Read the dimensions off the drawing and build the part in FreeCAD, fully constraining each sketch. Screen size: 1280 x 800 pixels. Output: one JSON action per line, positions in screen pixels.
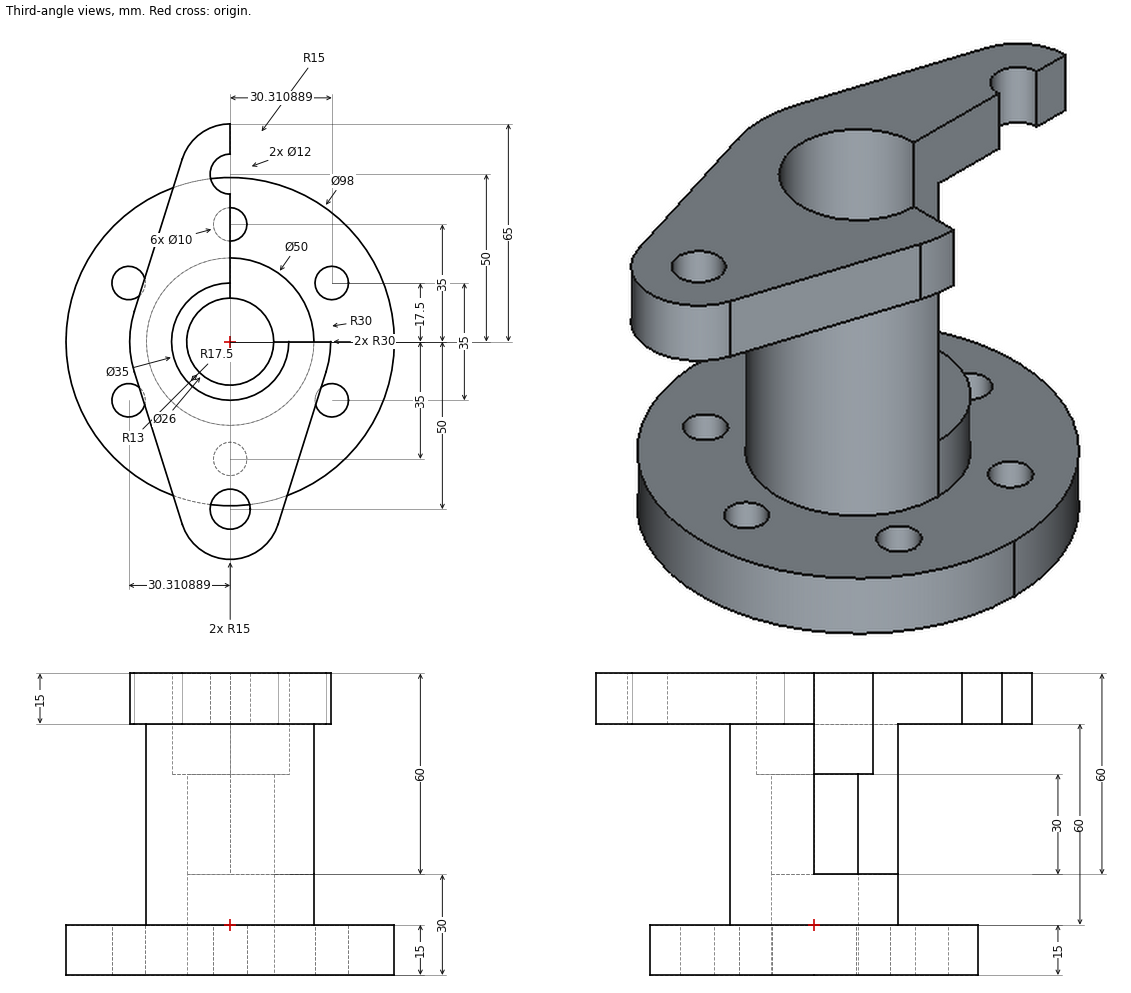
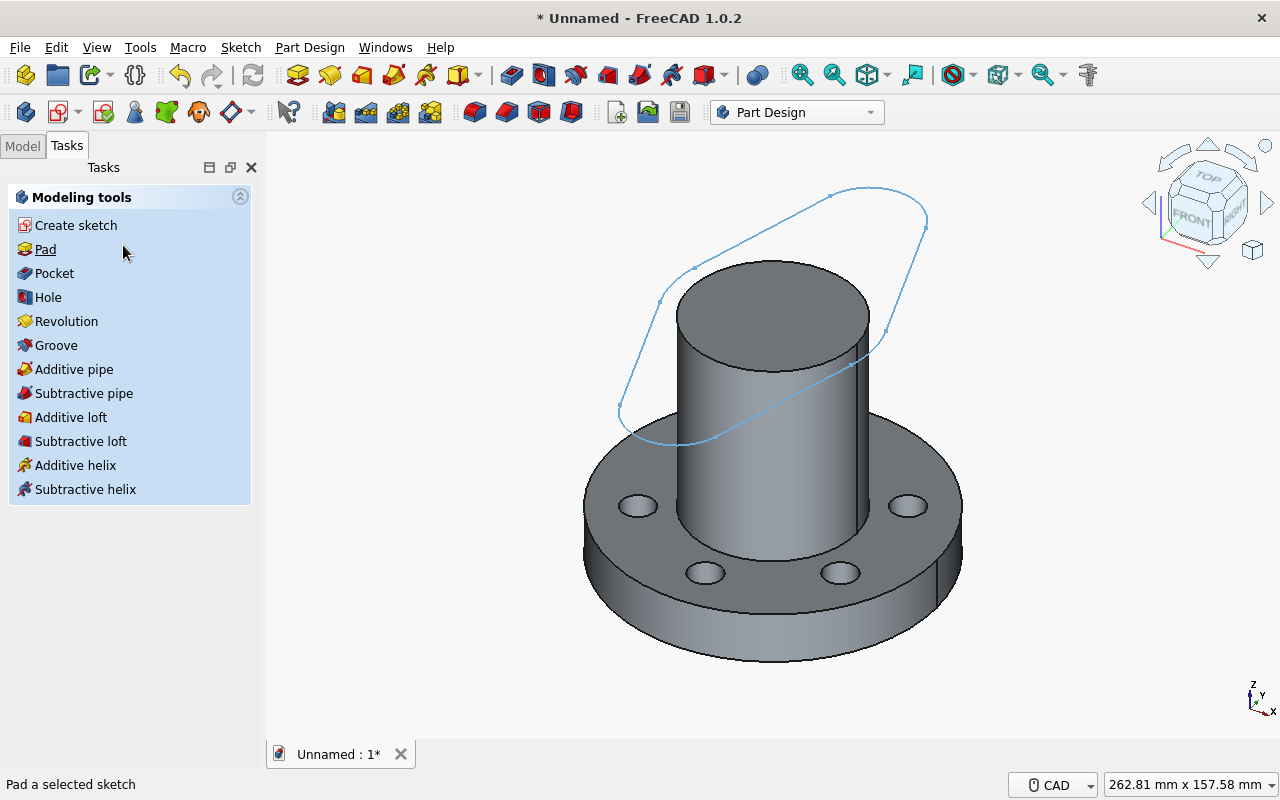
{"action": "left_click", "coordinate": [298, 76]}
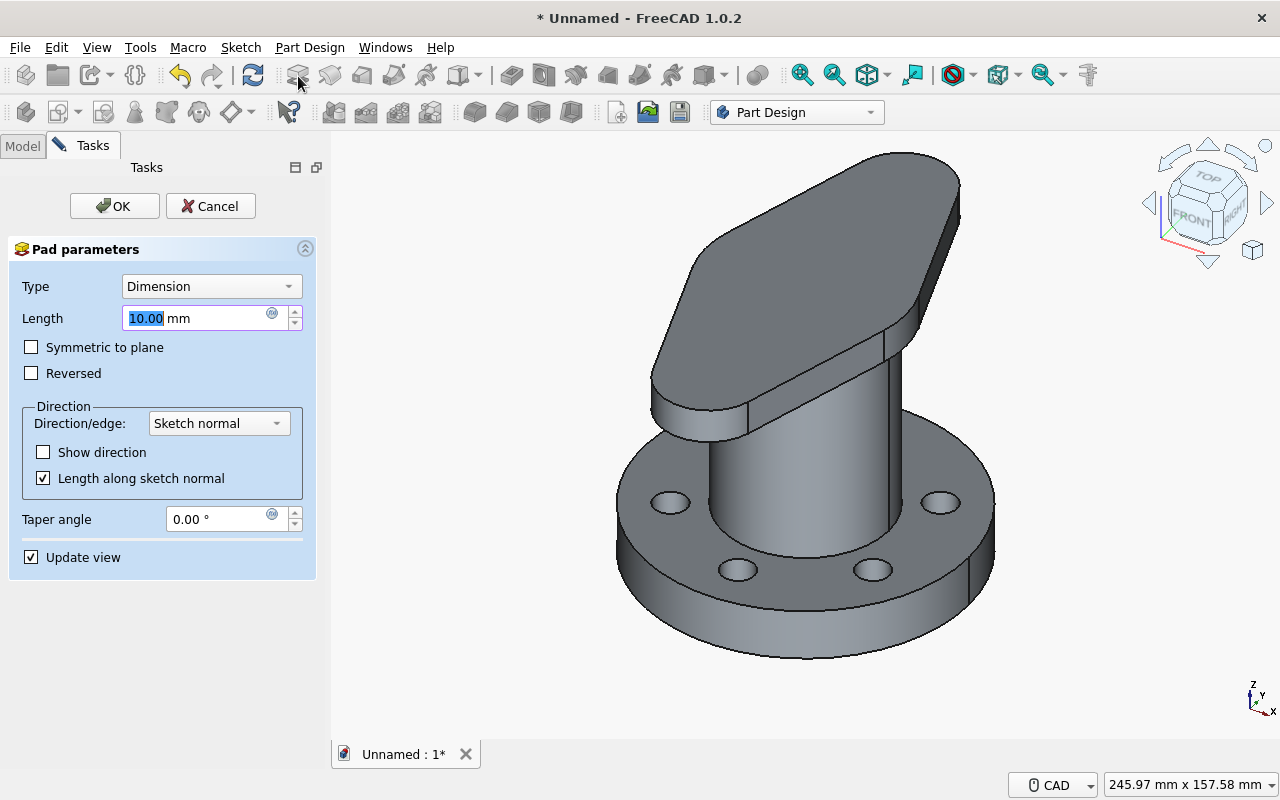
{"action": "type", "text": "15"}
{"action": "key", "text": "Tab"}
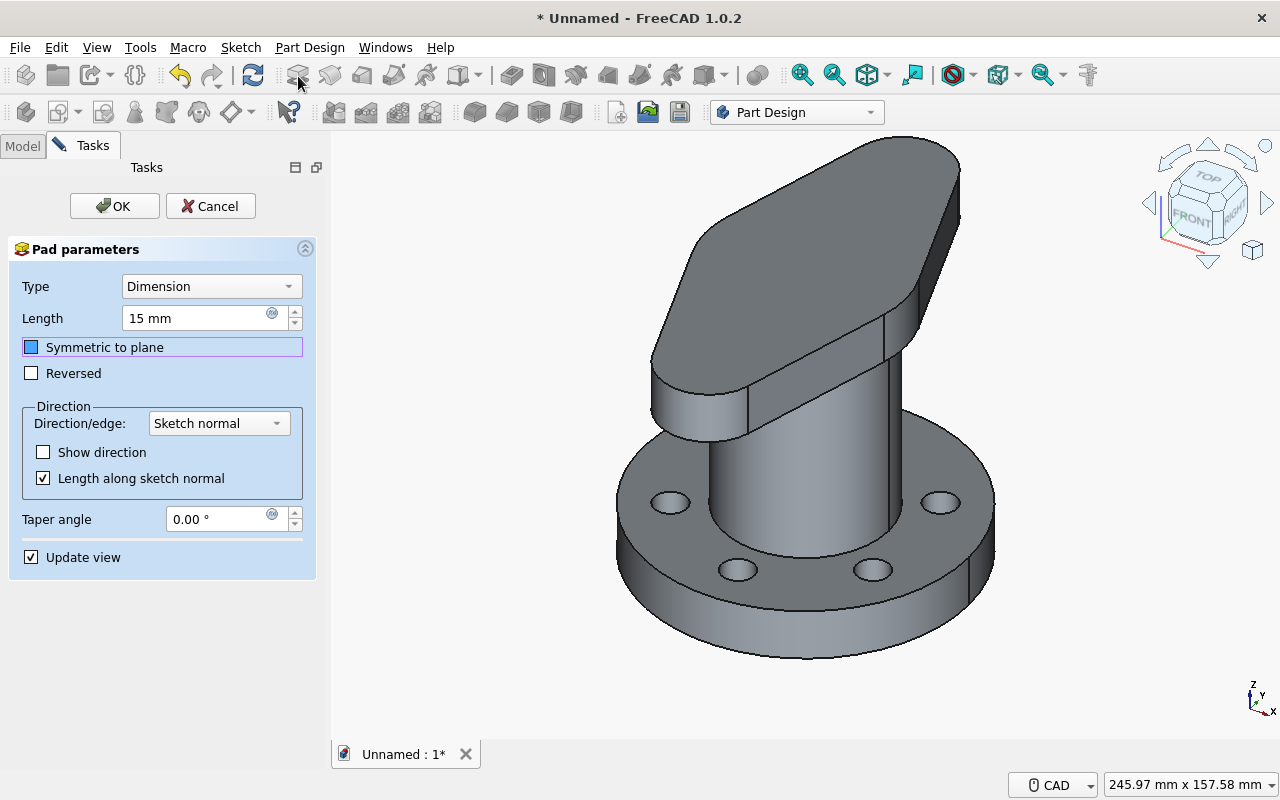
{"action": "left_click", "coordinate": [115, 206]}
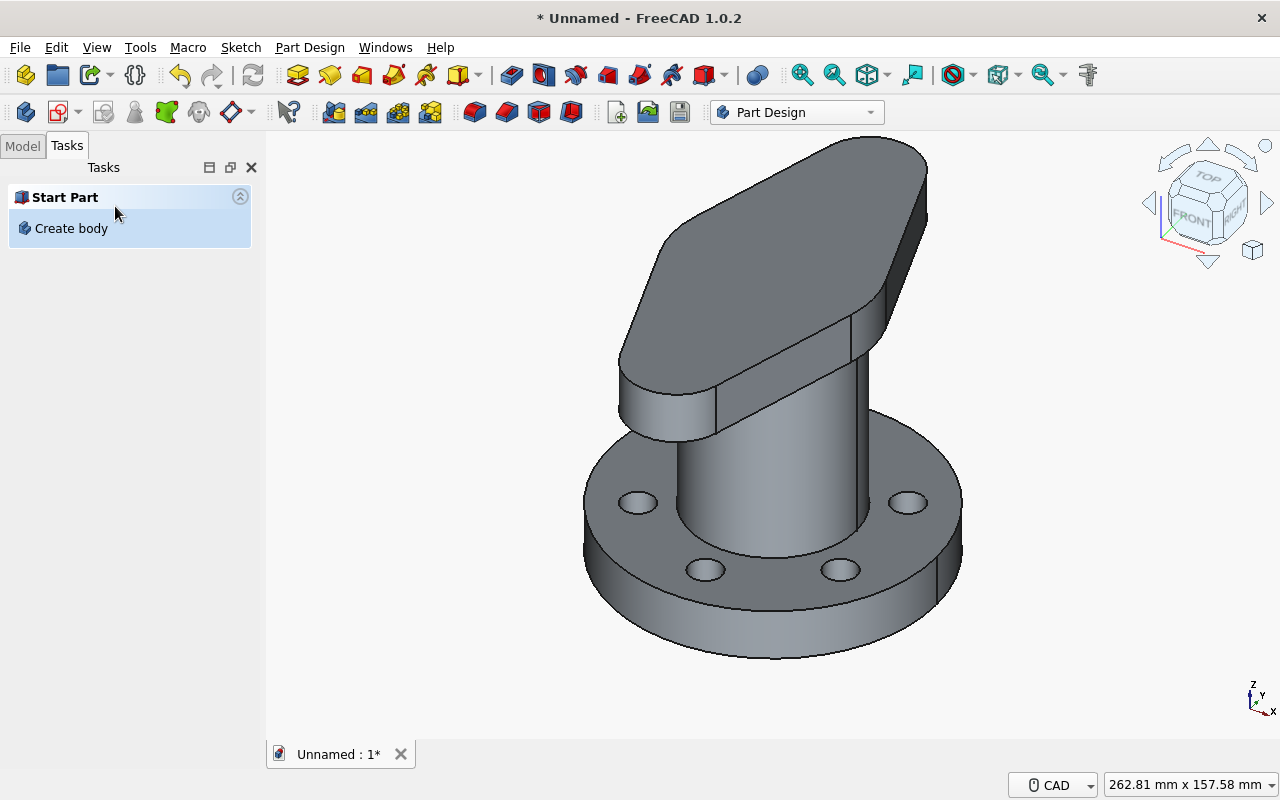
{"action": "left_click", "coordinate": [804, 76]}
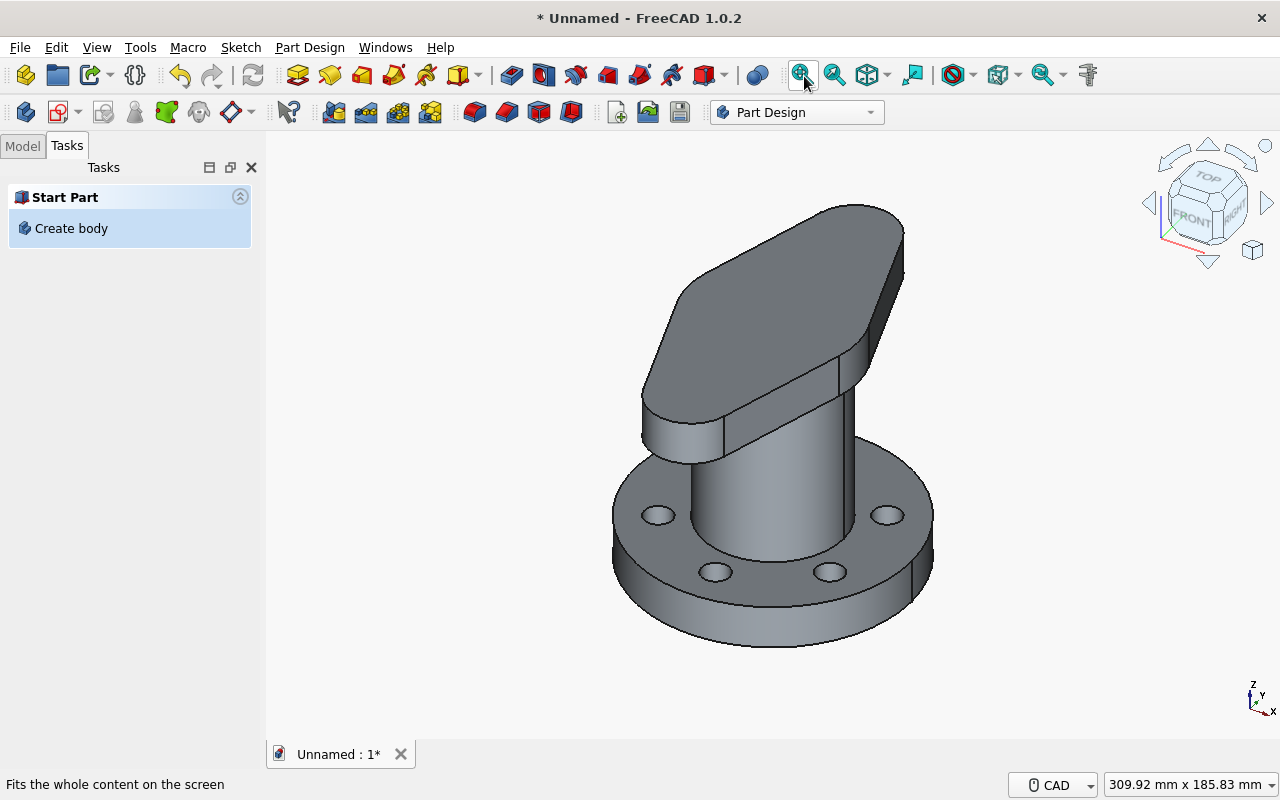
{"action": "left_click", "coordinate": [23, 145]}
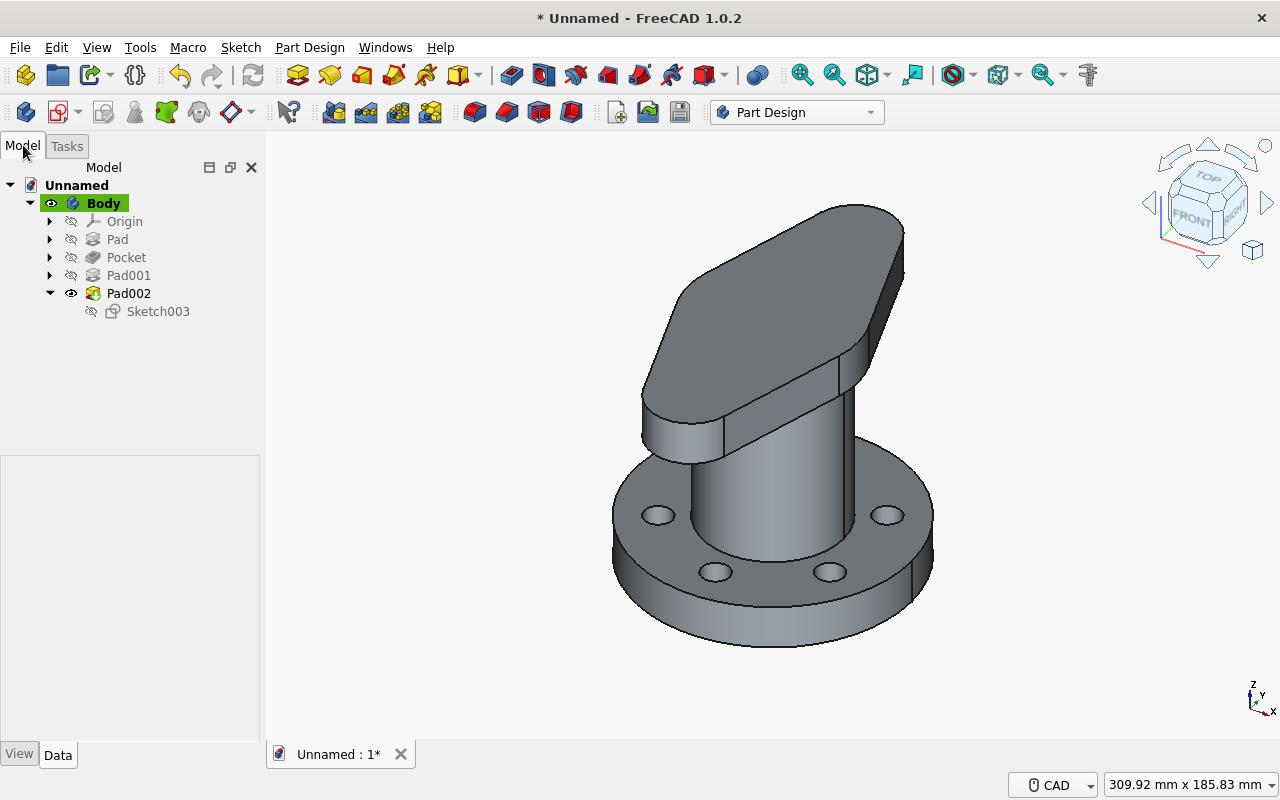
{"action": "left_click", "coordinate": [50, 221]}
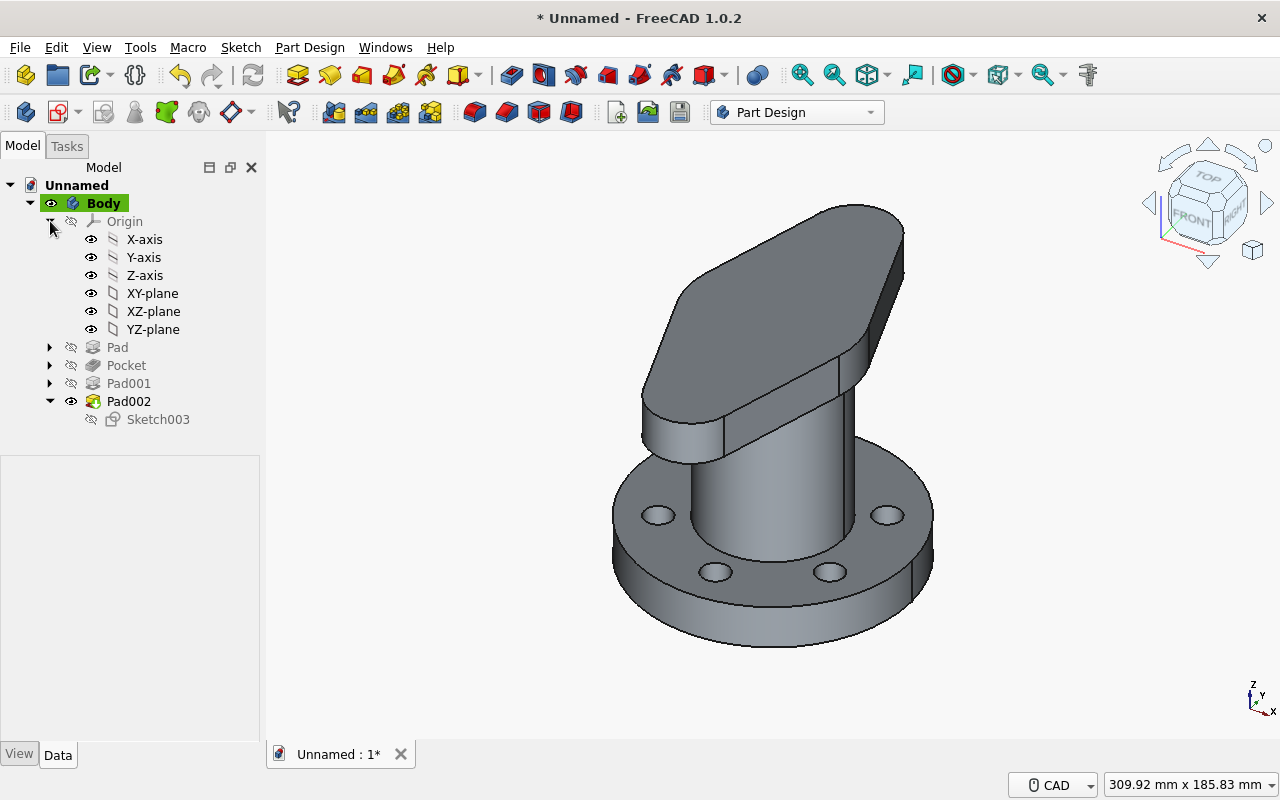
{"action": "left_click", "coordinate": [136, 293]}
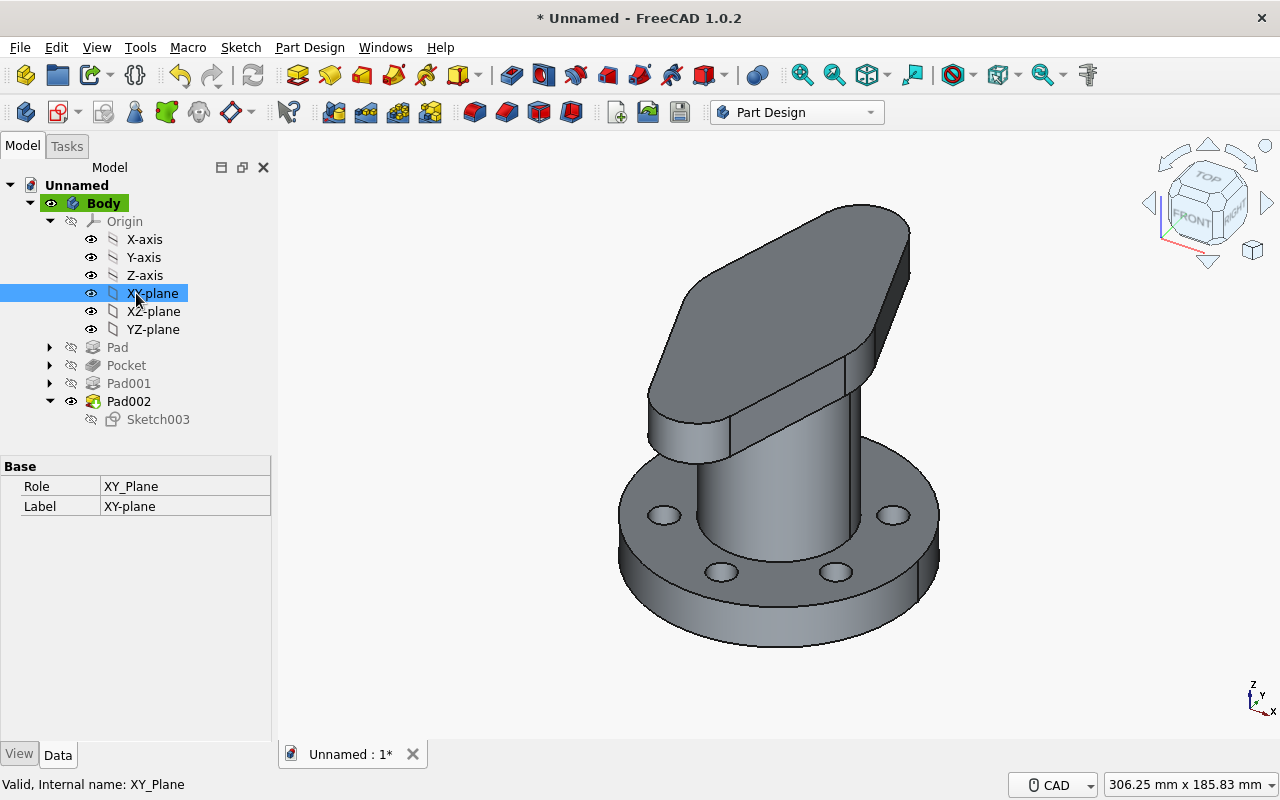
{"action": "left_click", "coordinate": [232, 112]}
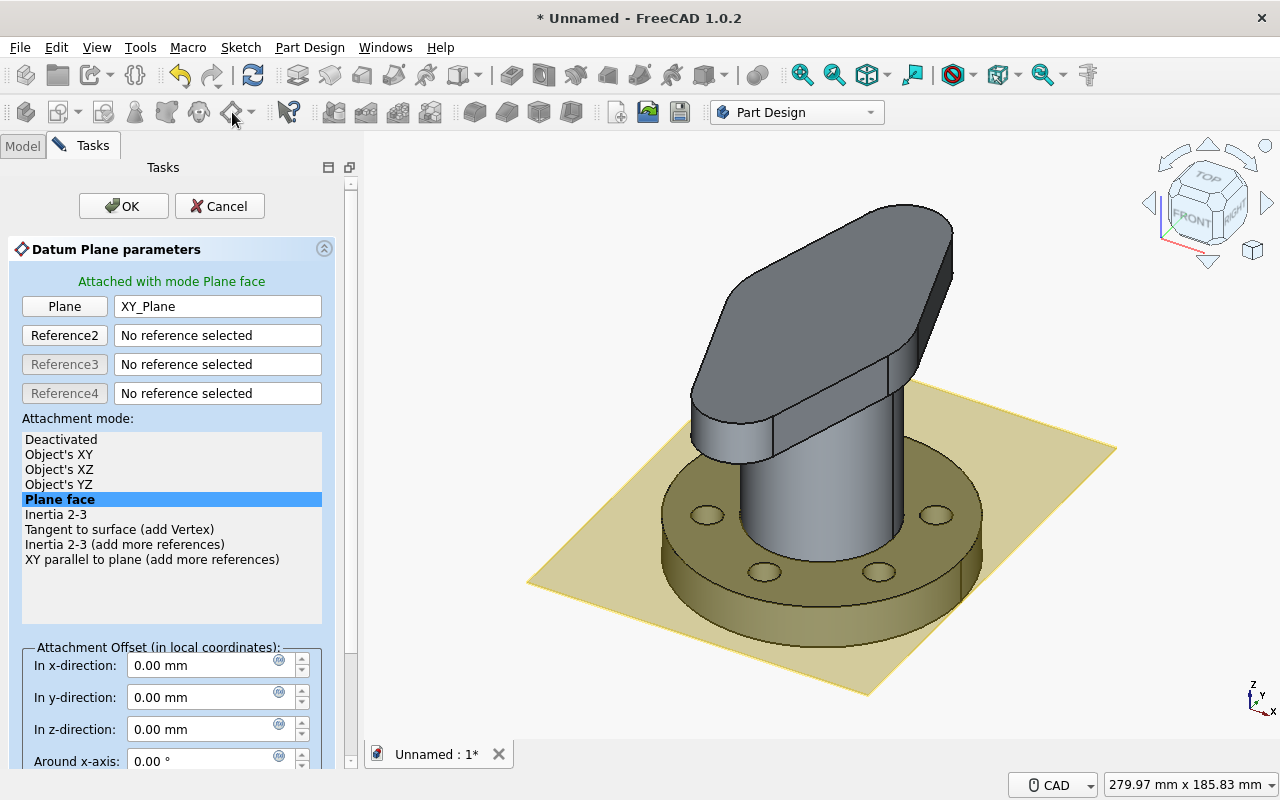
{"action": "triple_click", "coordinate": [210, 729]}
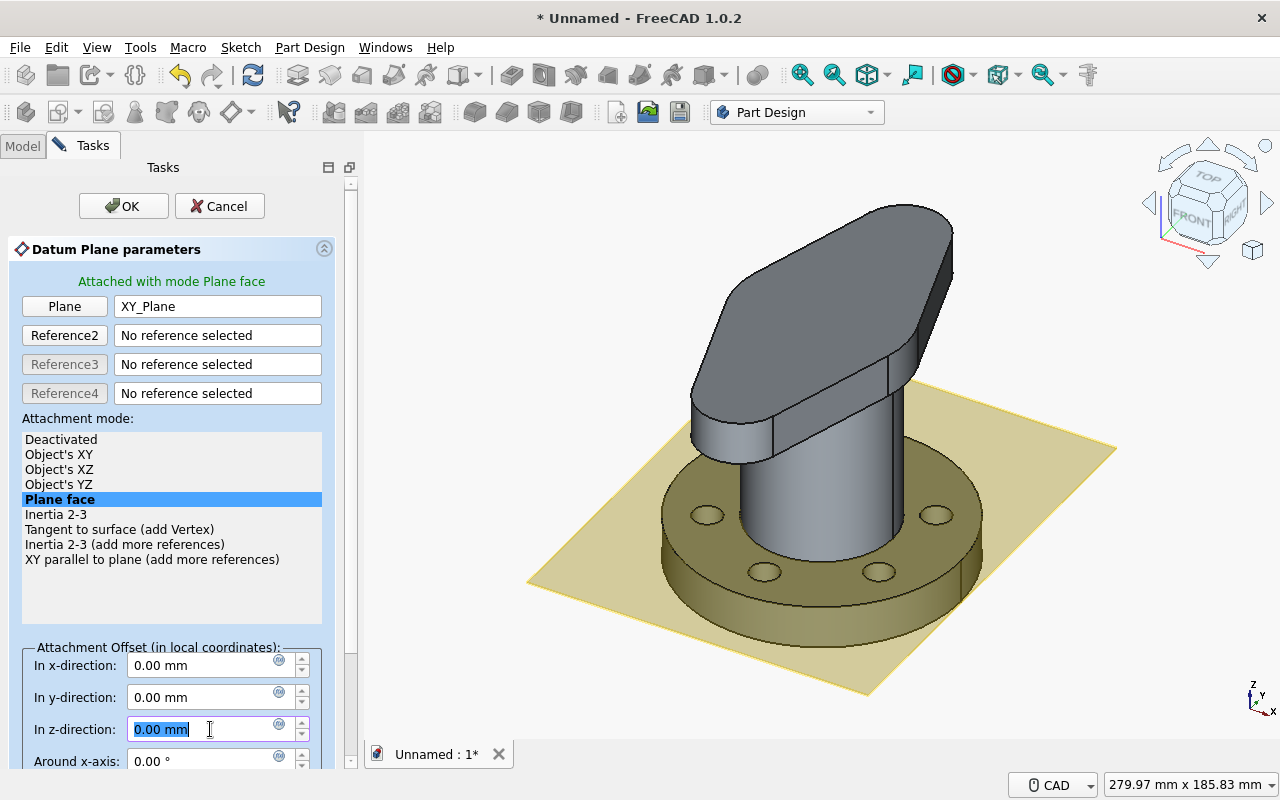
{"action": "type", "text": "15"}
{"action": "key", "text": "Tab"}